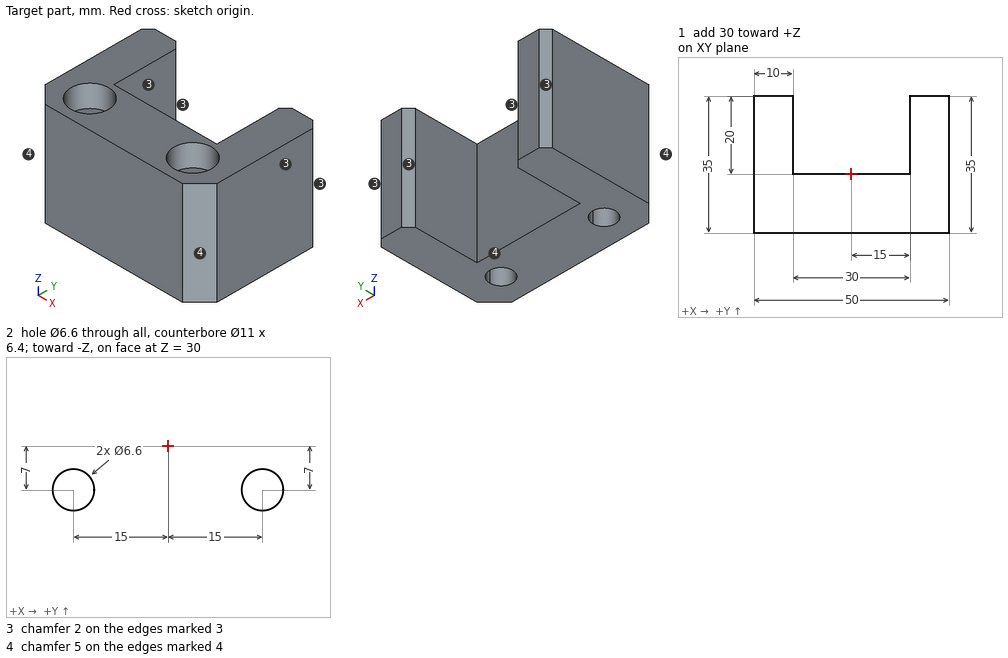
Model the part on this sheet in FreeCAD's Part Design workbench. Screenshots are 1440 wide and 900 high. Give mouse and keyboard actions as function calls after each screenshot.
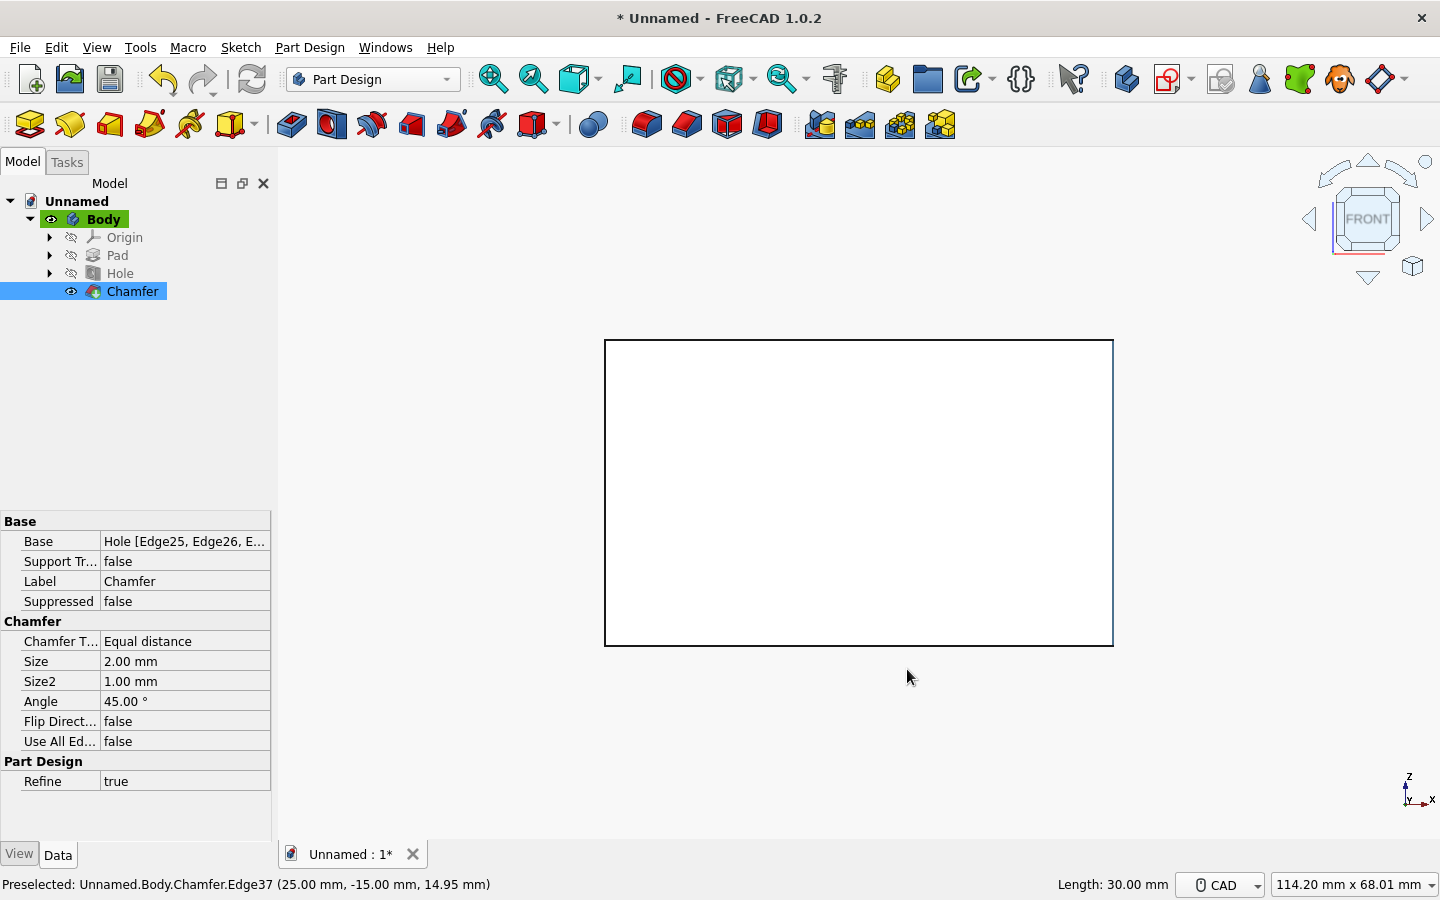
click(494, 80)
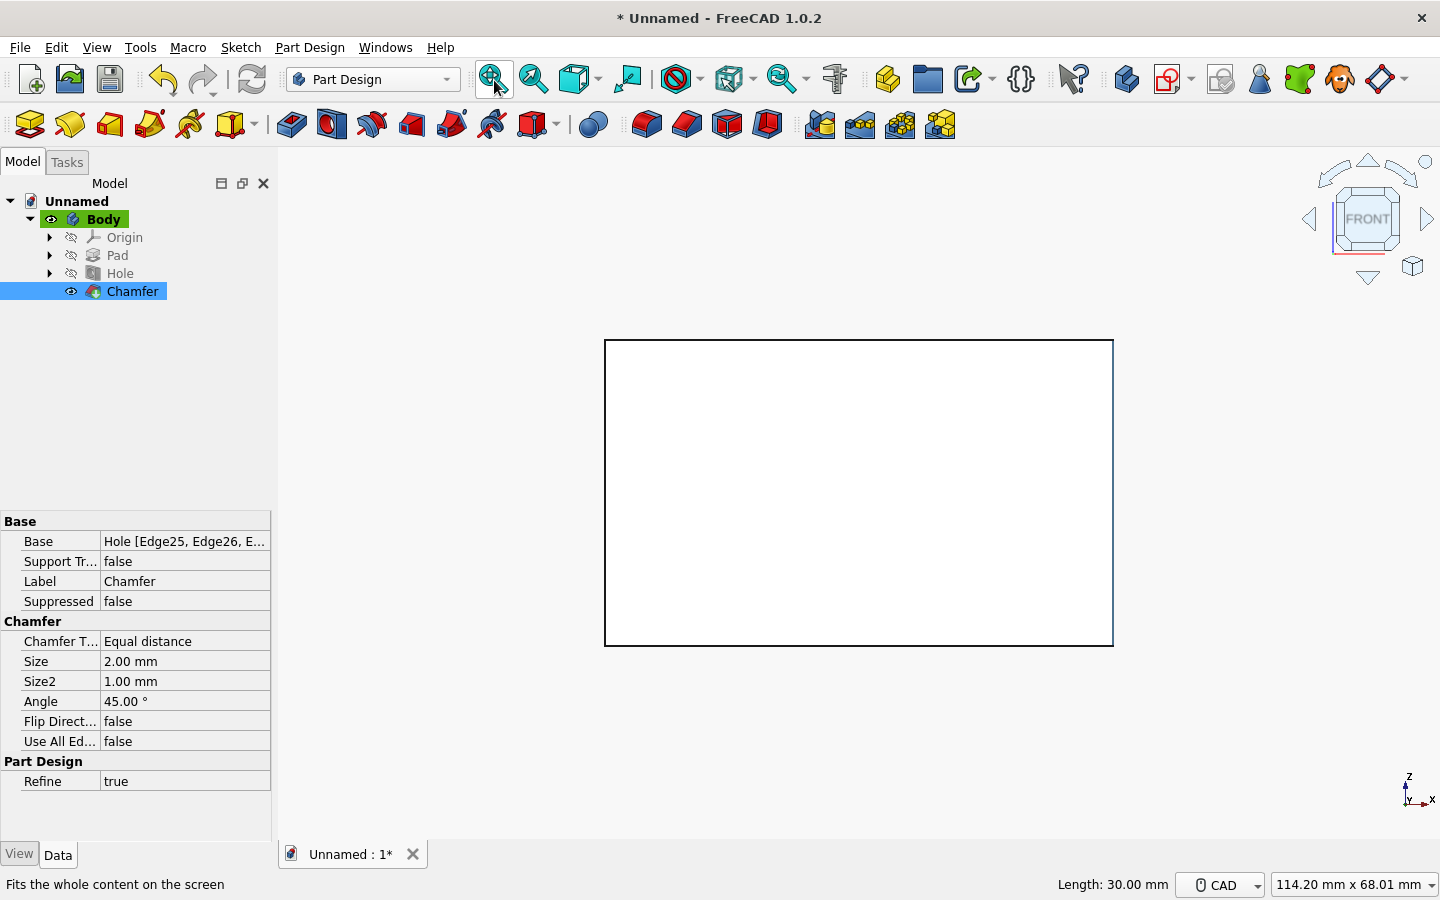
click(605, 492, ctrl)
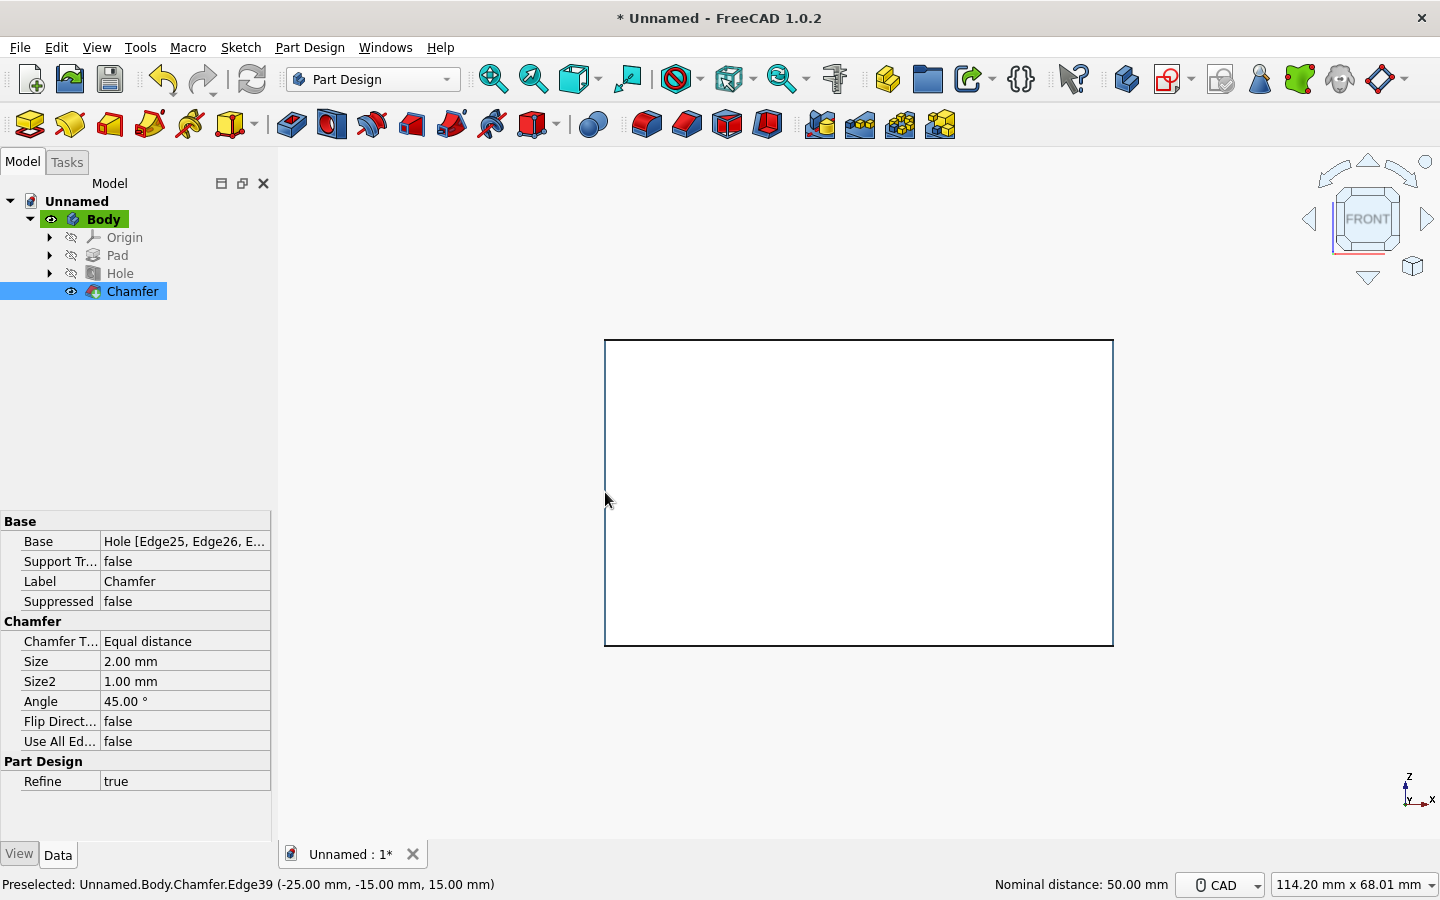
click(688, 124)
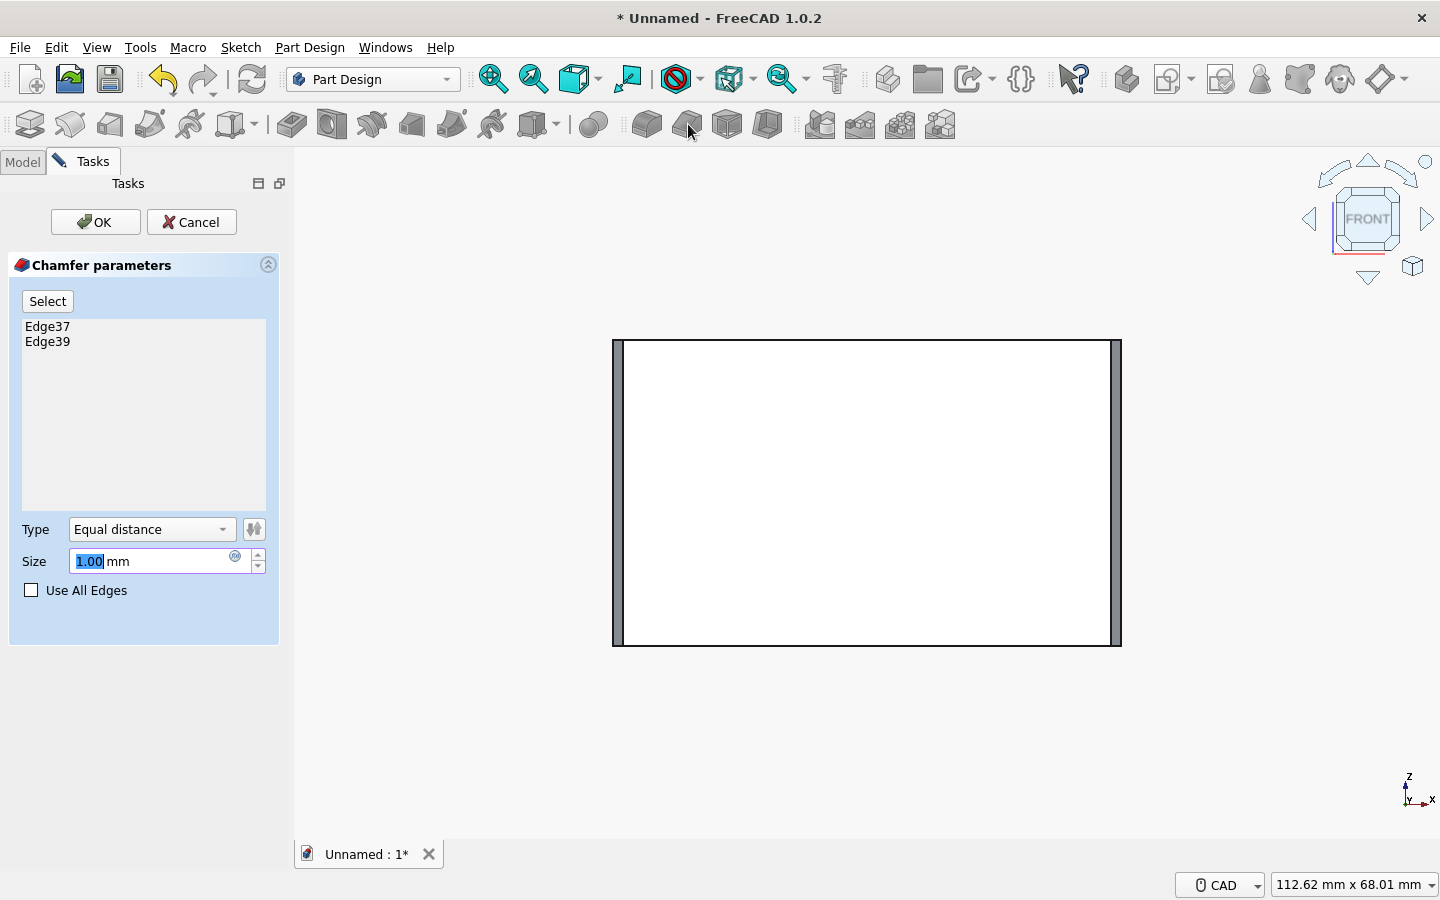
text(5)
key(Tab)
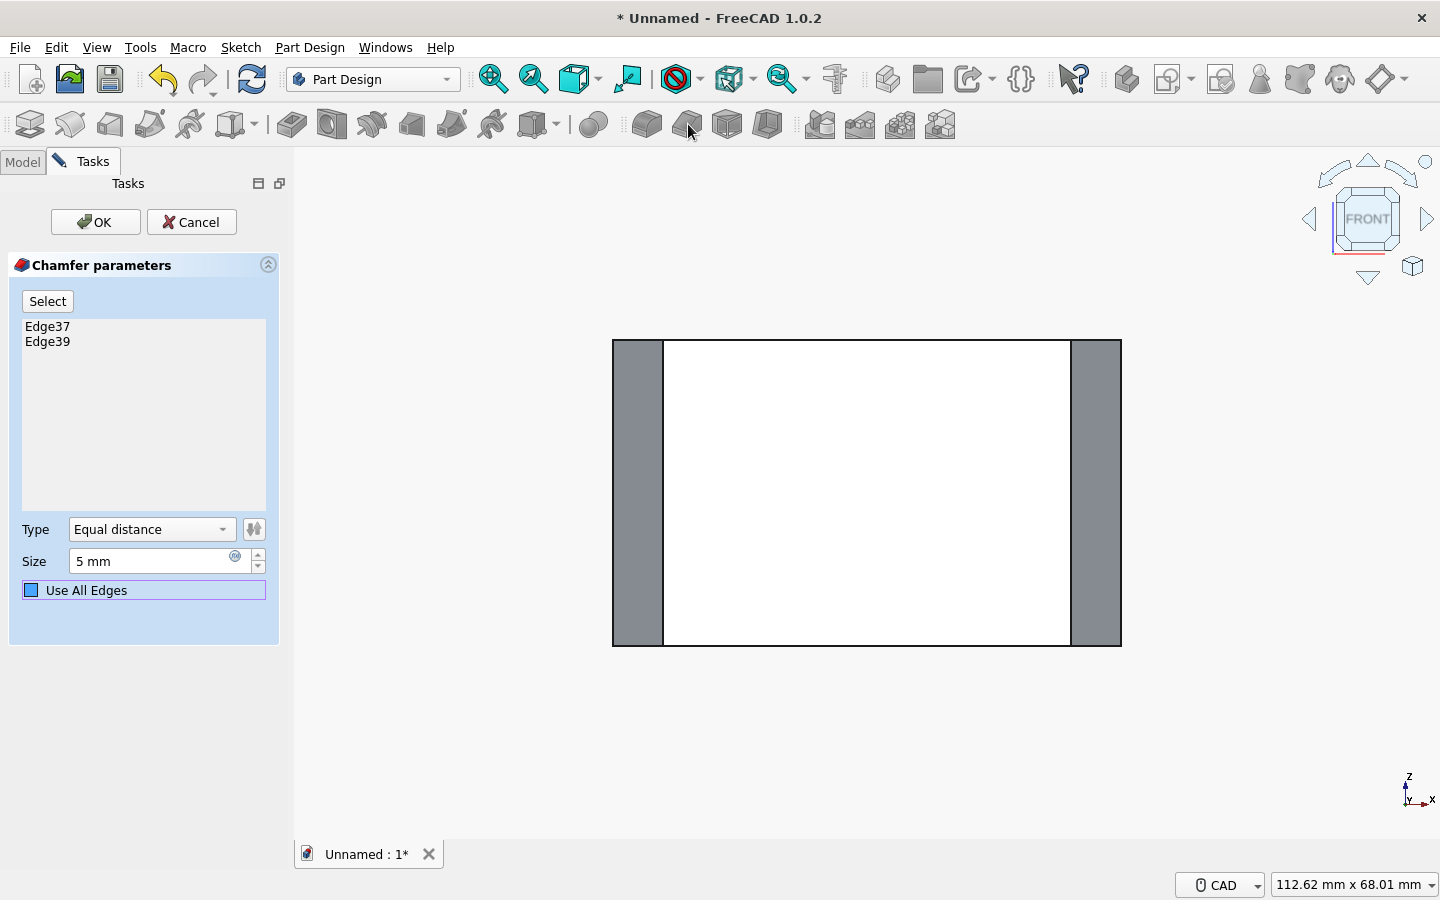
click(96, 222)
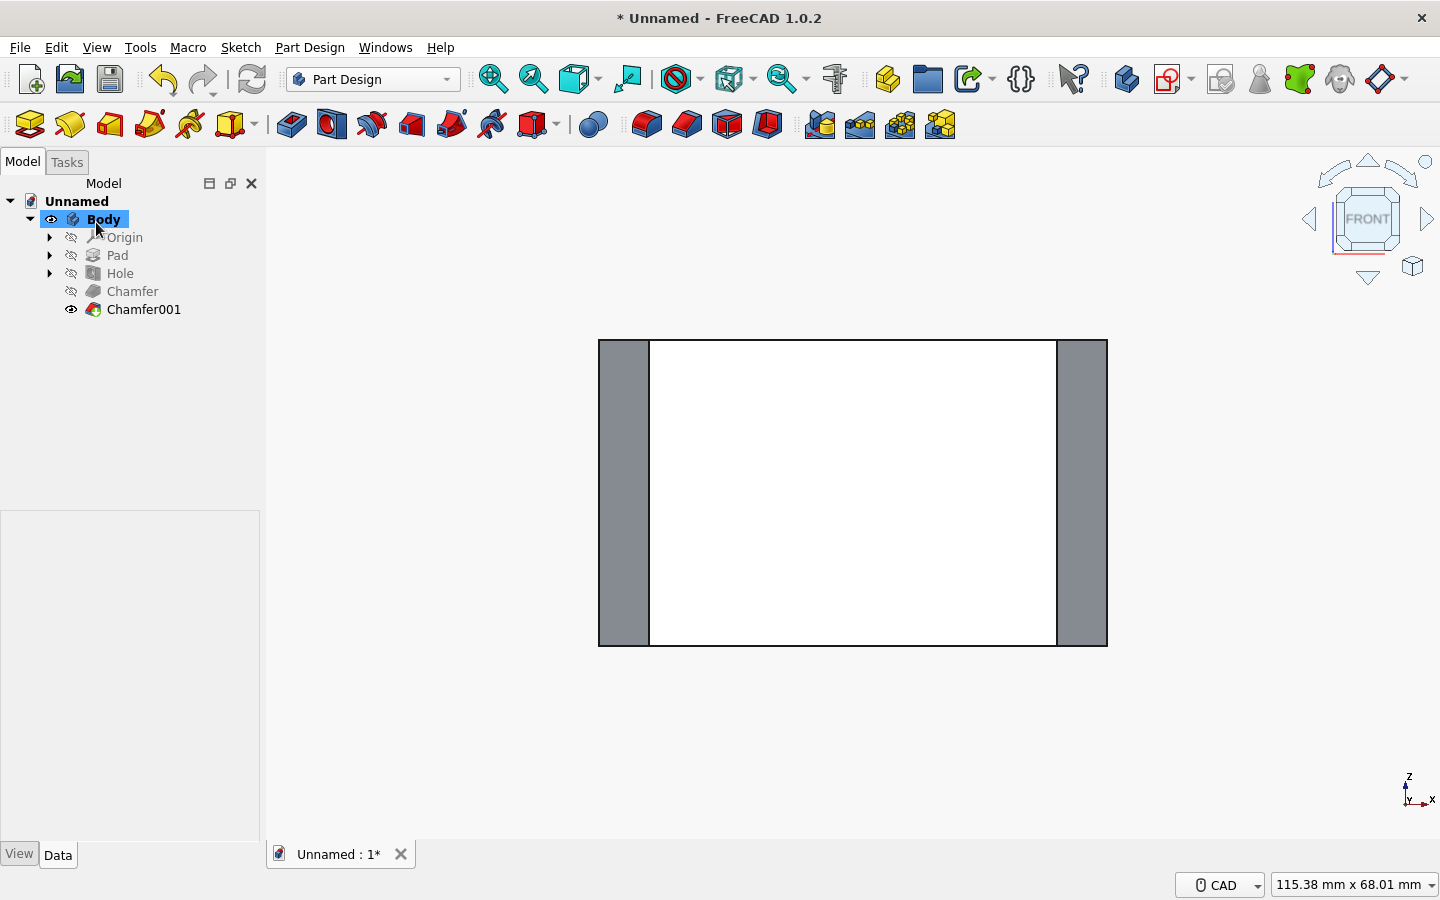
key(0)